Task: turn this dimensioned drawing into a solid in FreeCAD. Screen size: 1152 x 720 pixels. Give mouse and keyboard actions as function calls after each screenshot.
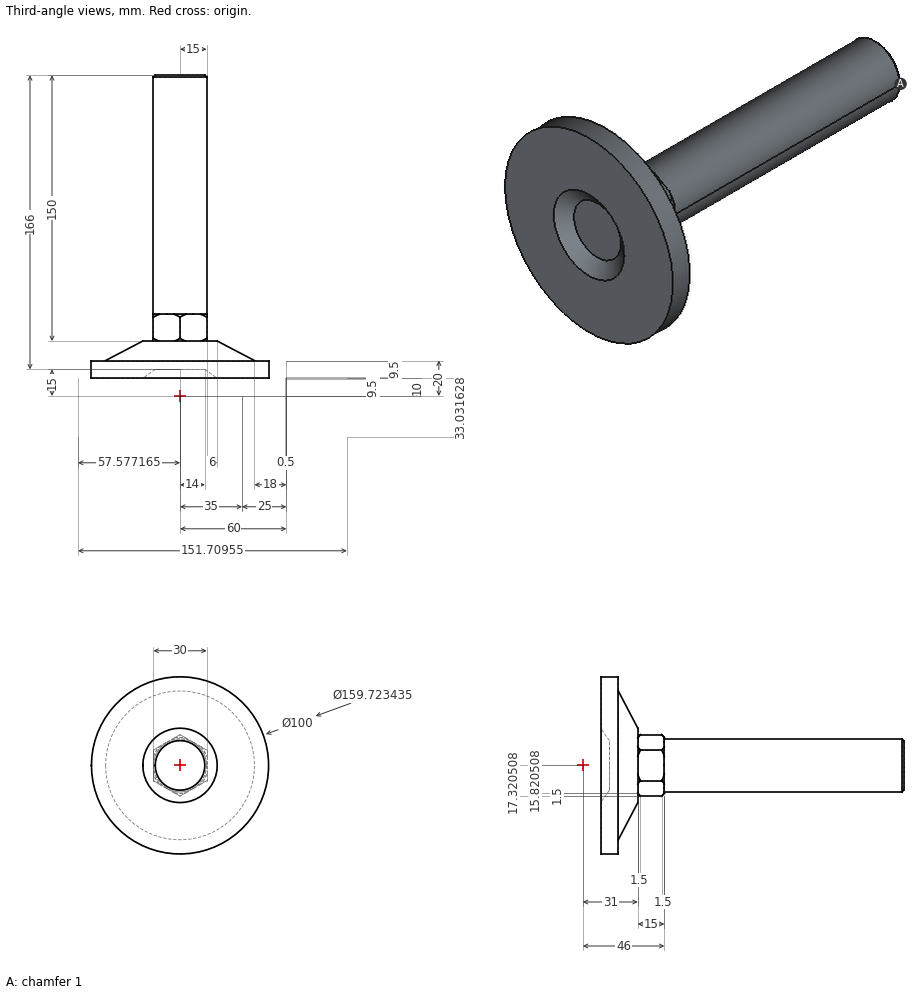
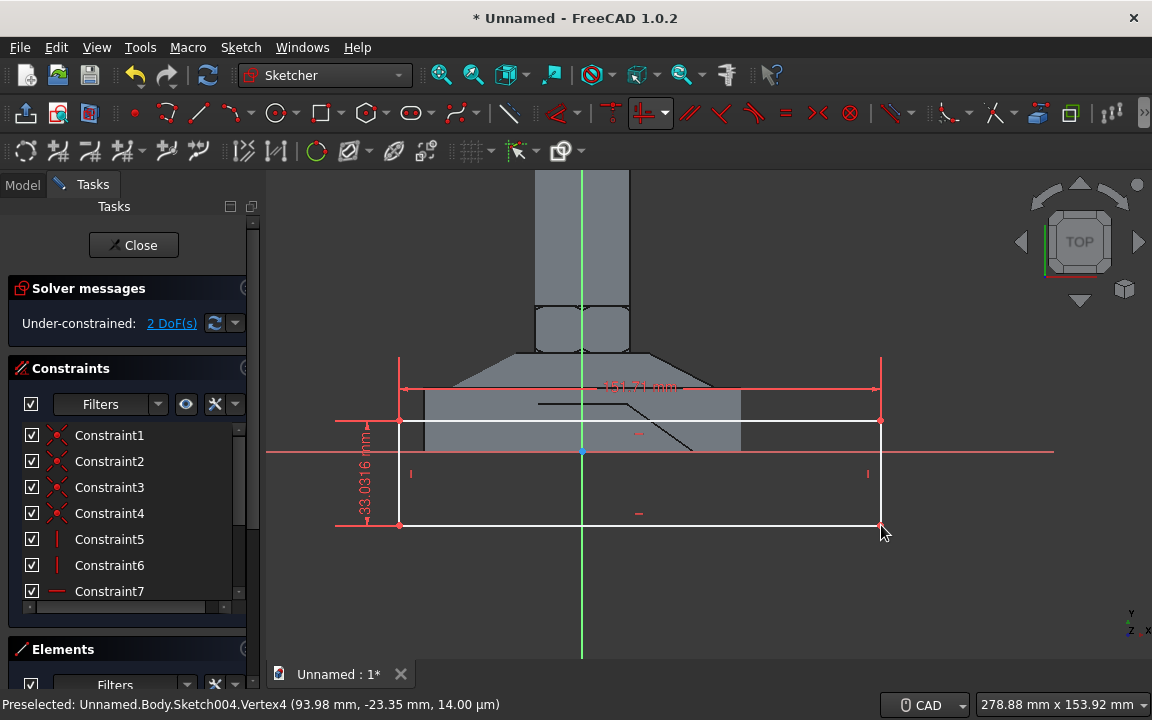
click(556, 114)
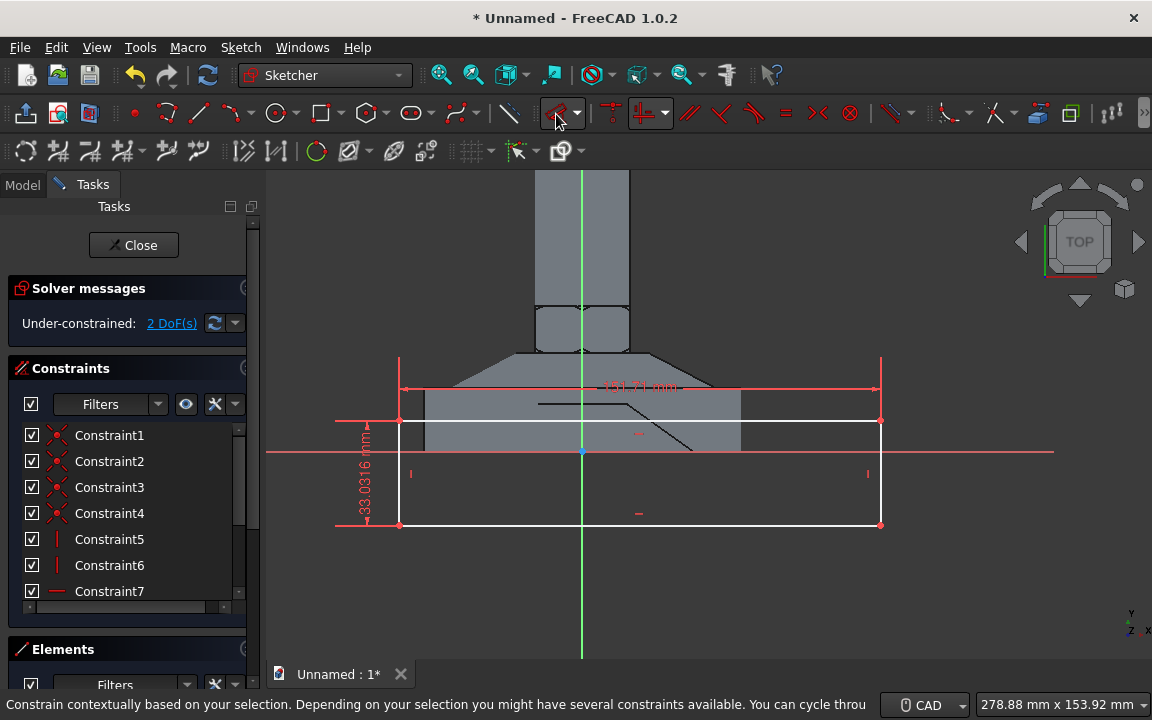
scroll(399, 421, up, 2)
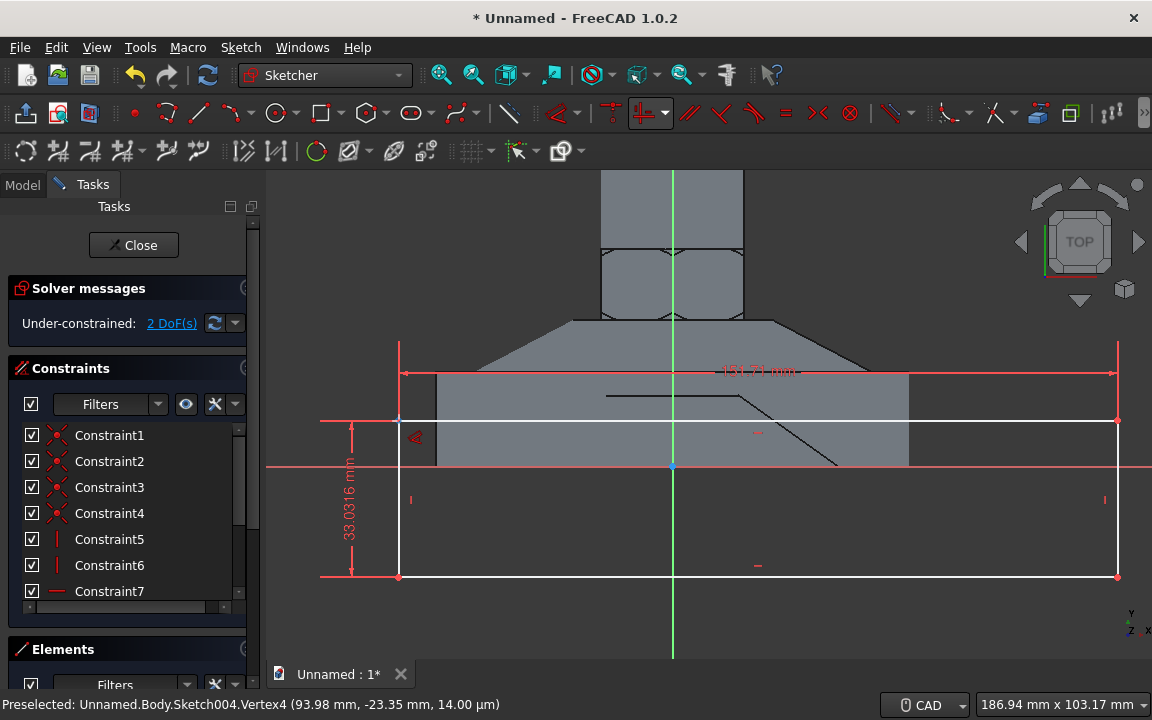
click(399, 421)
click(365, 444)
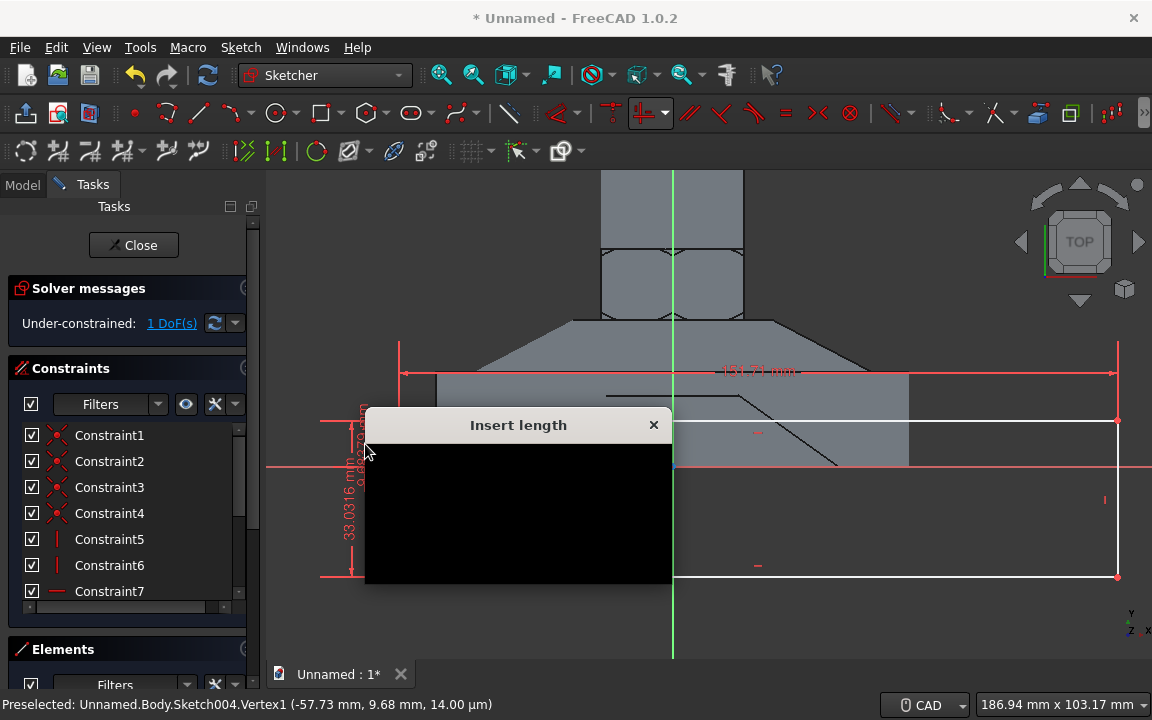
text(10)
key(Return)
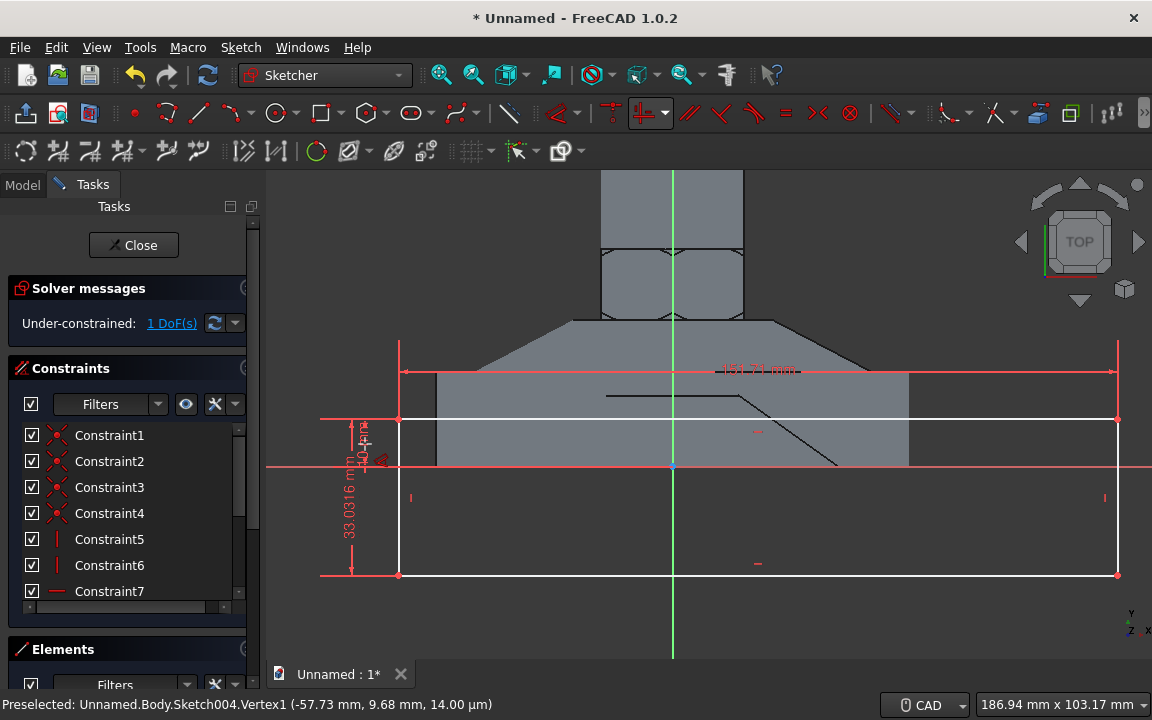
click(399, 419)
click(536, 385)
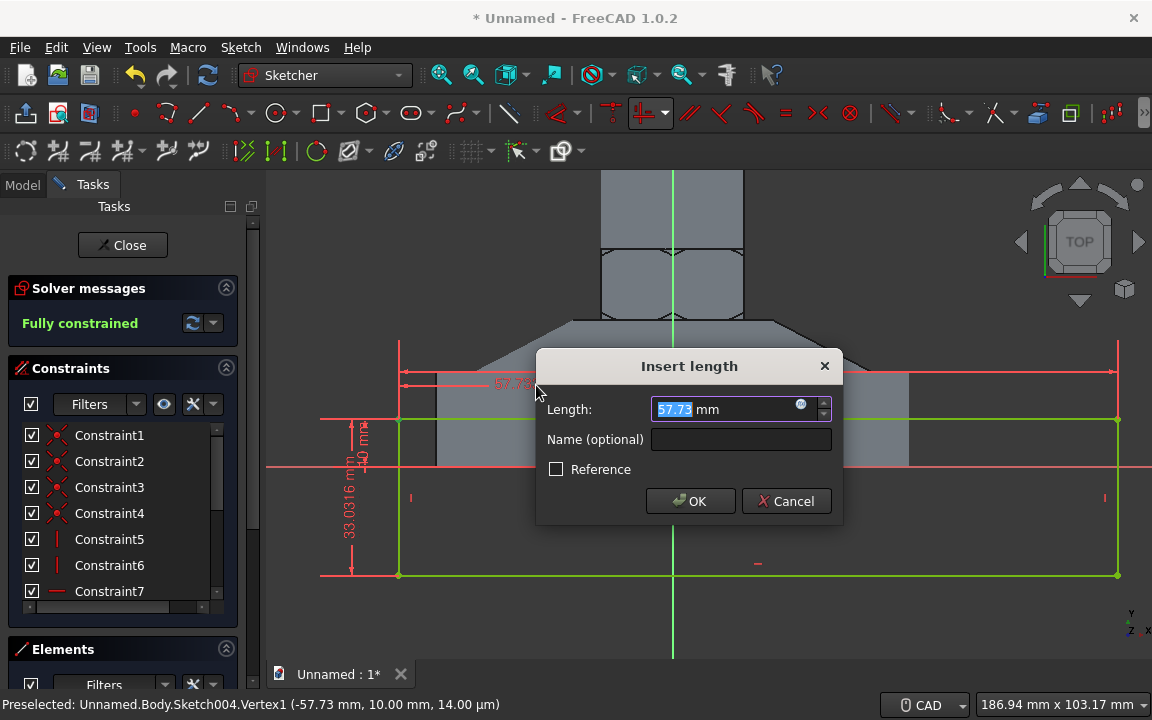
text(57.577165)
key(Return)
key(Escape)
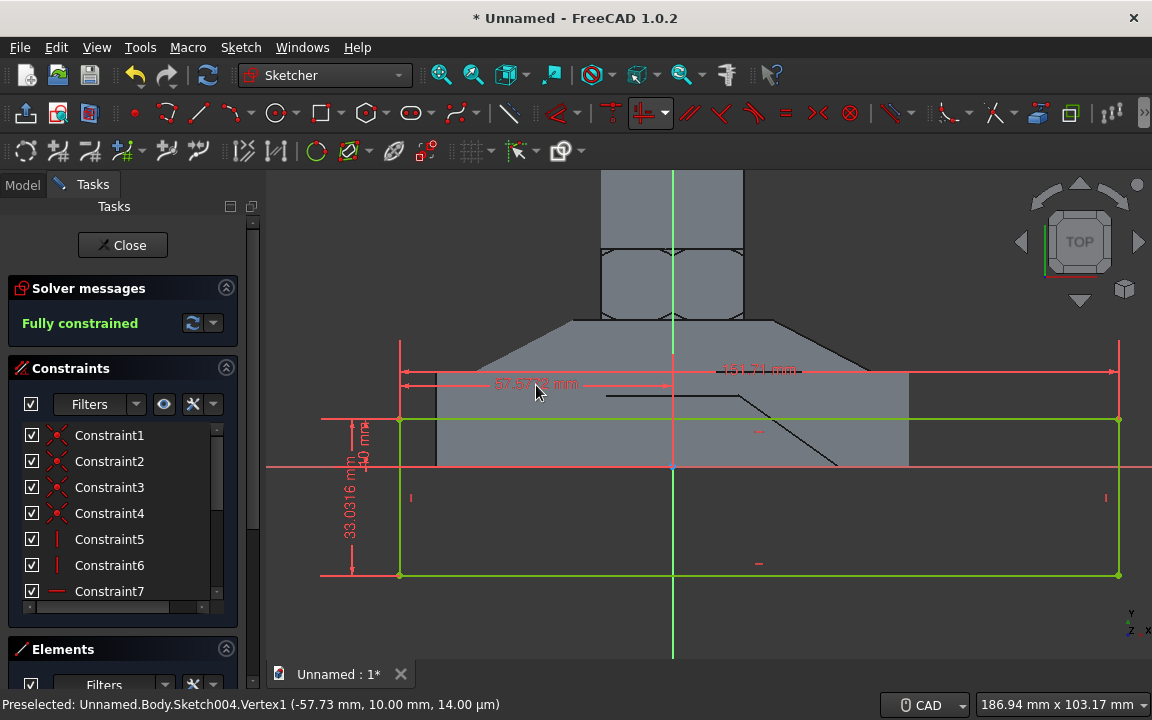
click(123, 245)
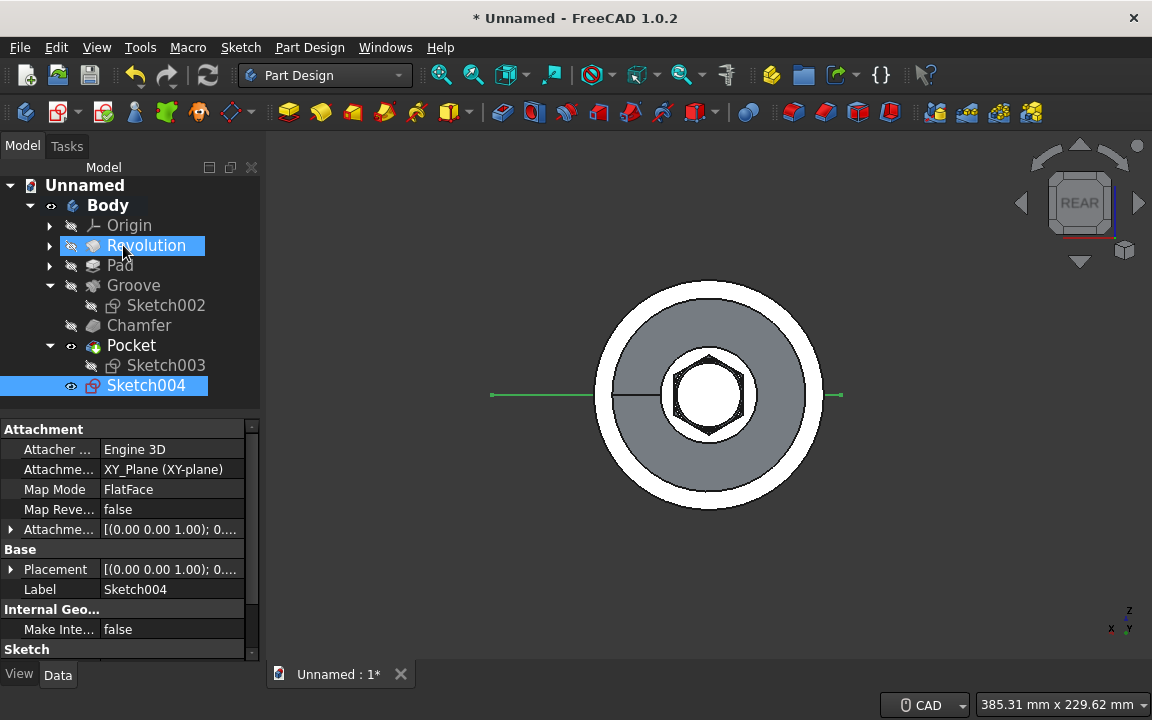
click(504, 112)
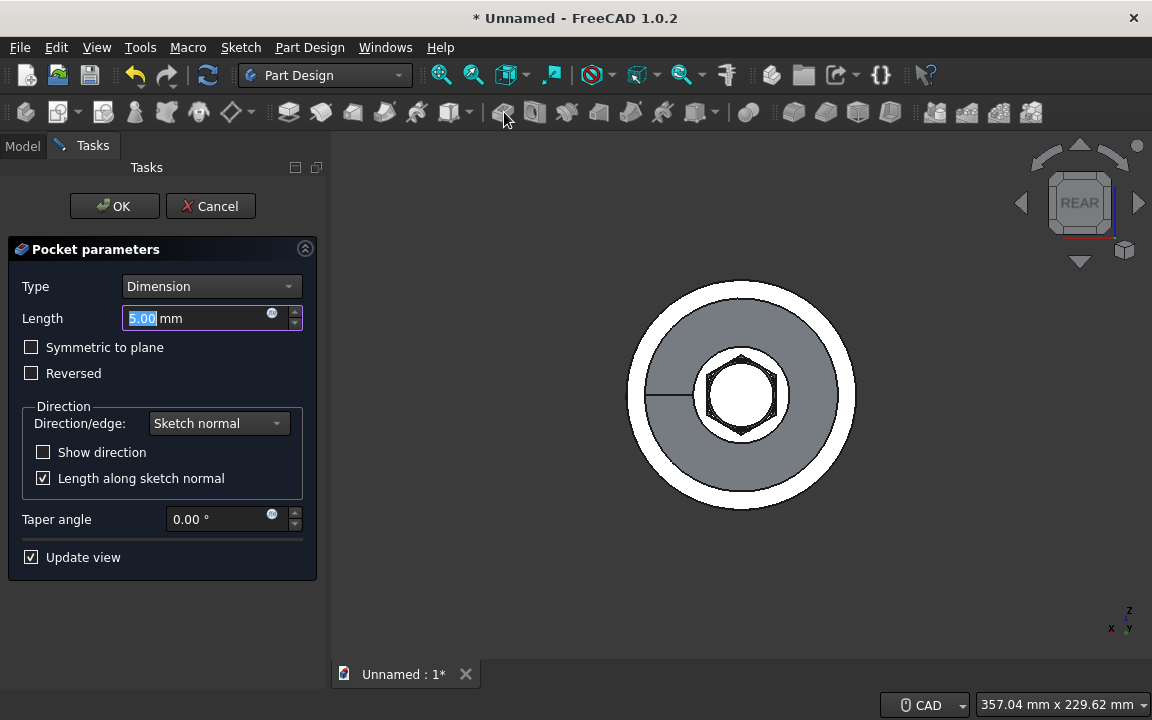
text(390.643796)
key(Tab)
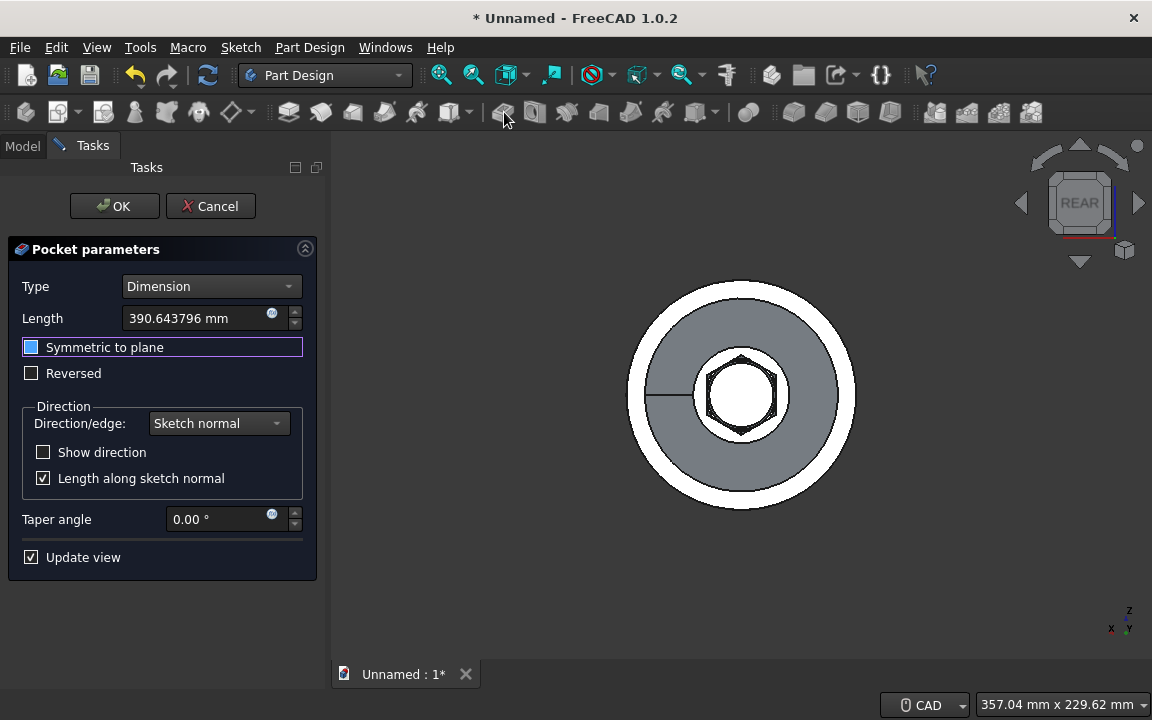
click(30, 347)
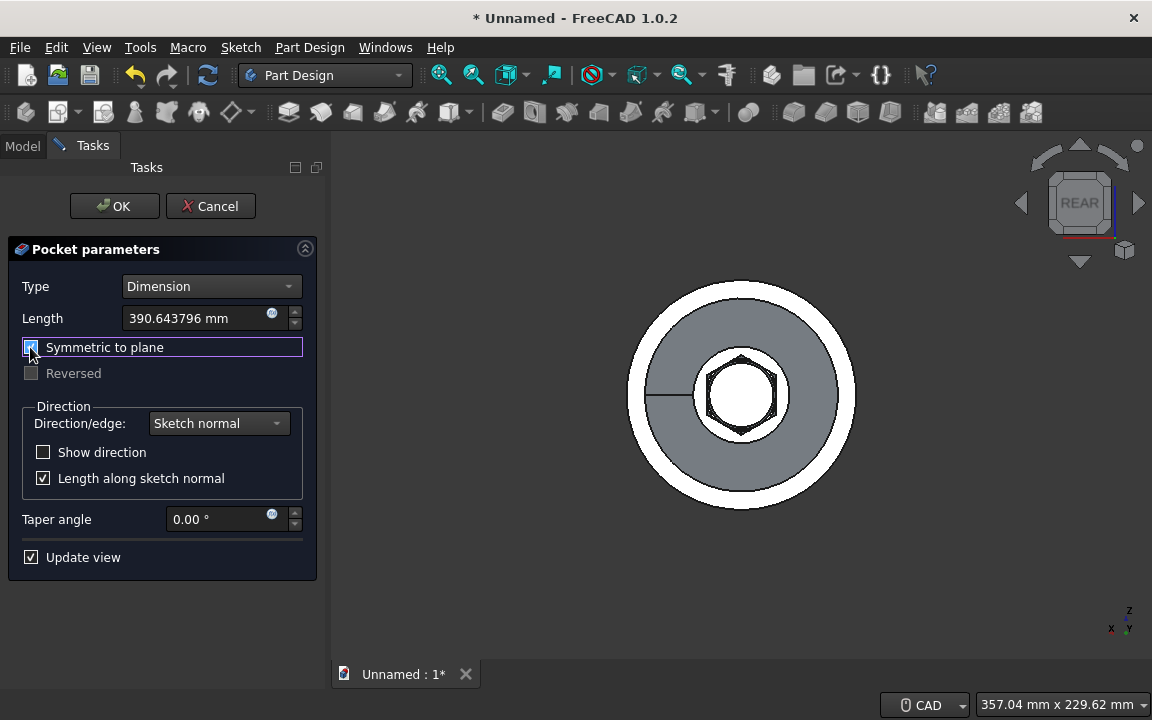
click(115, 206)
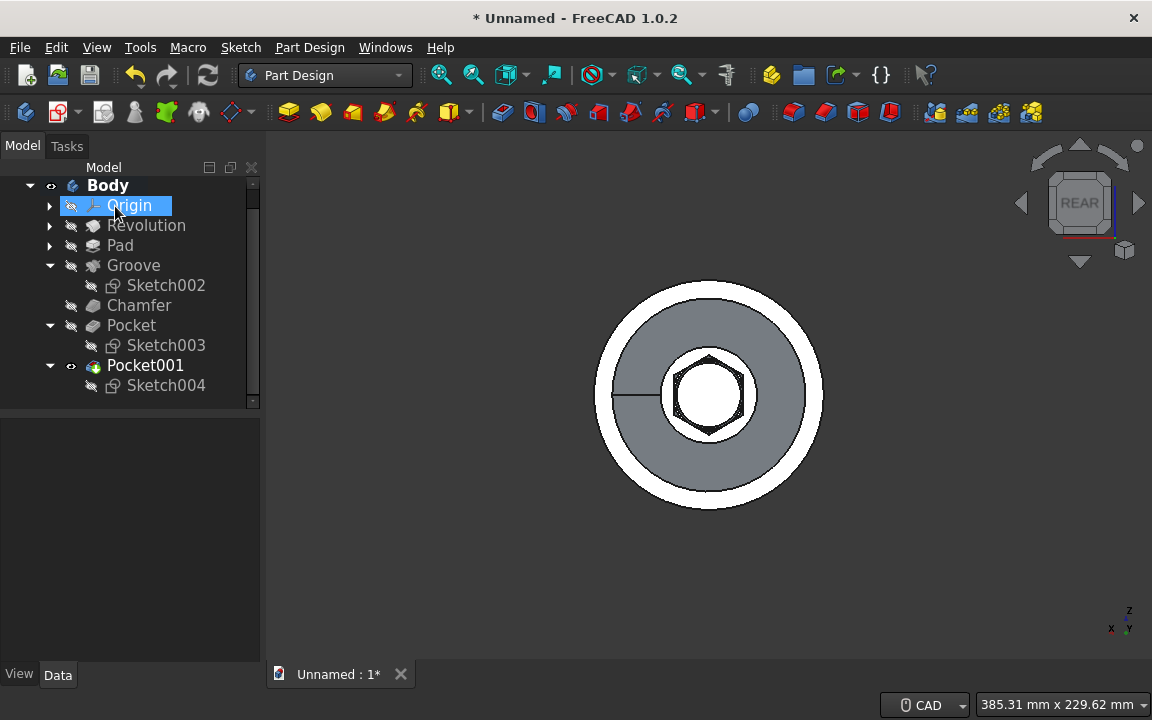
key(0)